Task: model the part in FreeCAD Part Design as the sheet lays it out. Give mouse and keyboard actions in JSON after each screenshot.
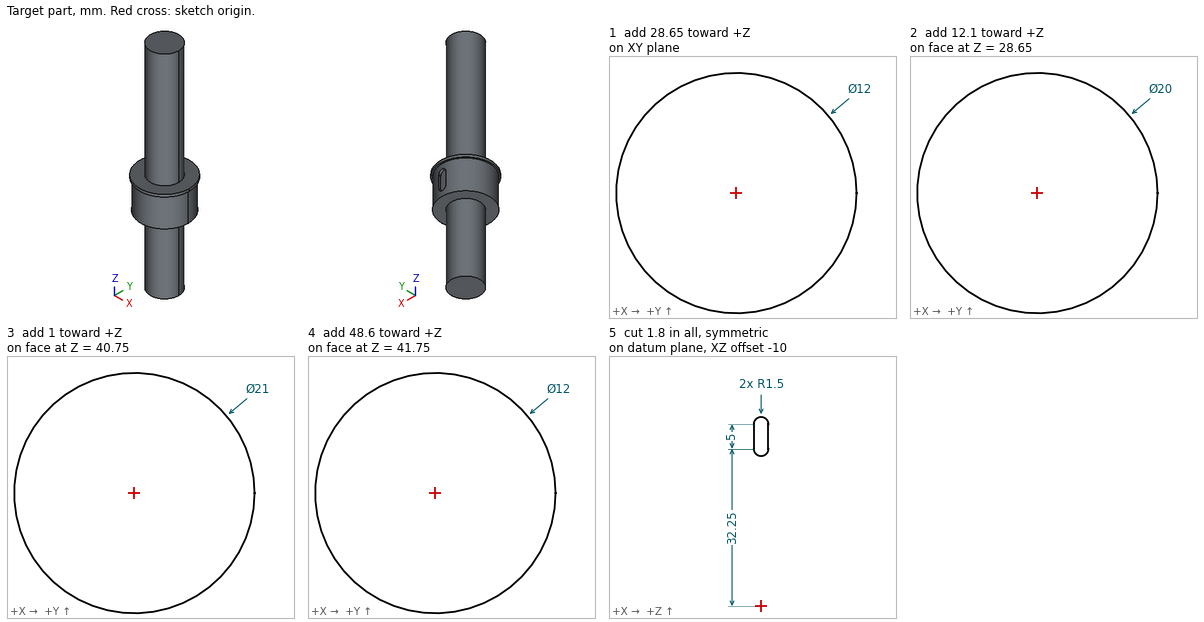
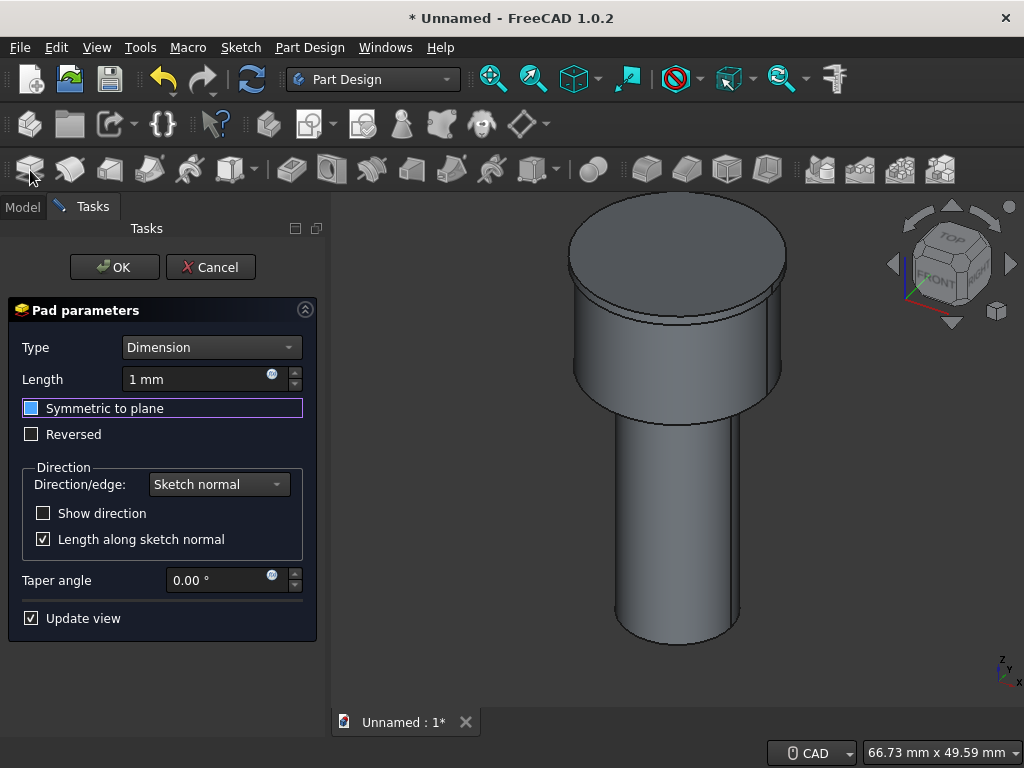
{"action": "left_click", "coordinate": [115, 267]}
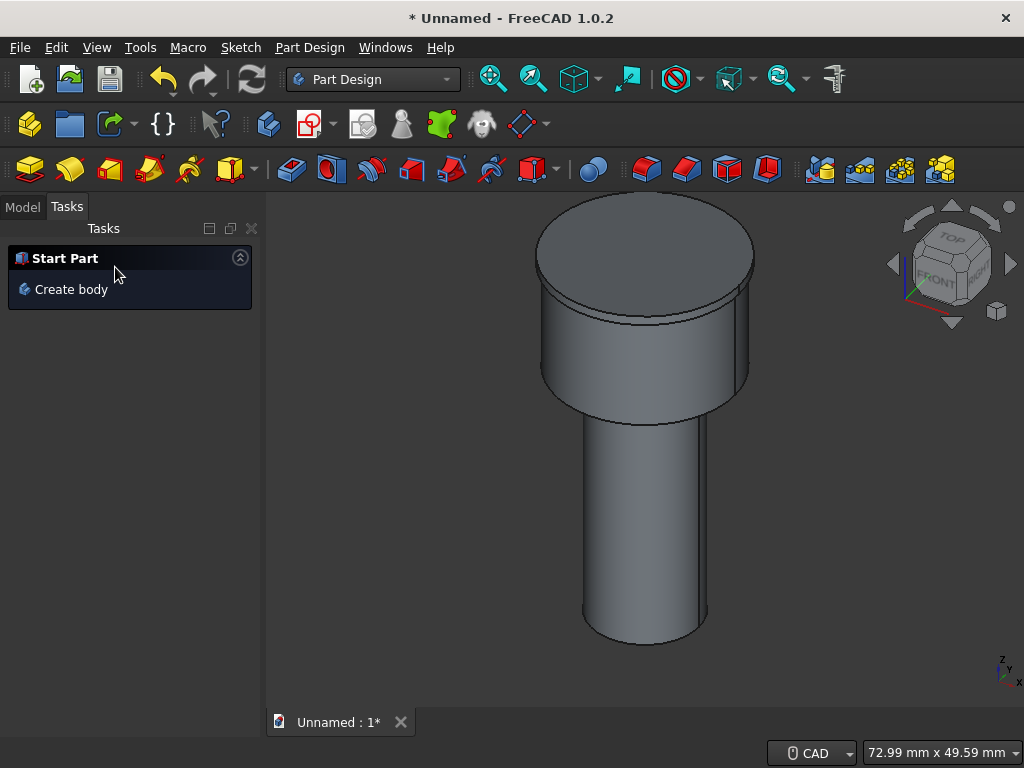
{"action": "left_click", "coordinate": [494, 80]}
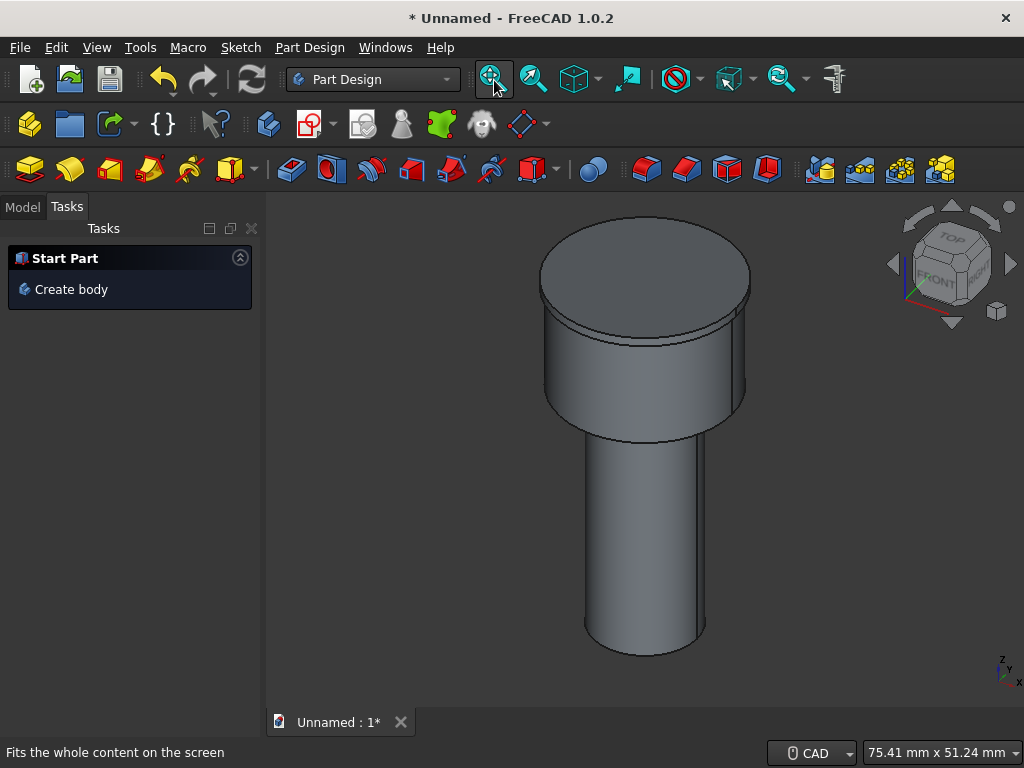
{"action": "left_click", "coordinate": [645, 277]}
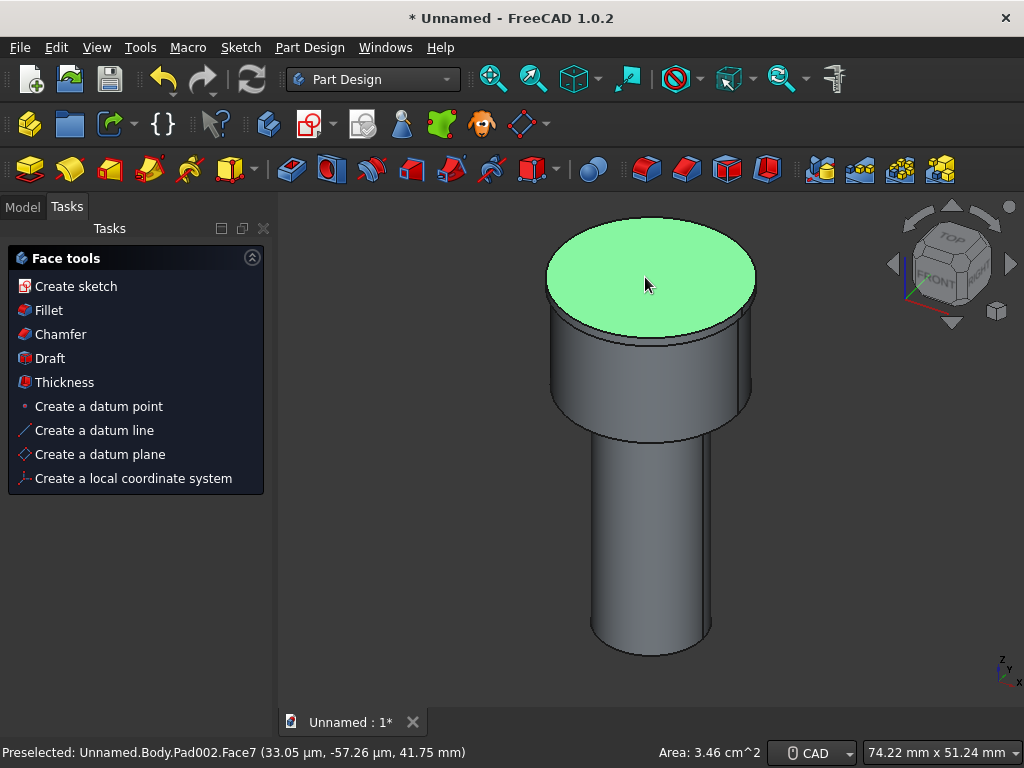
{"action": "left_click", "coordinate": [310, 124]}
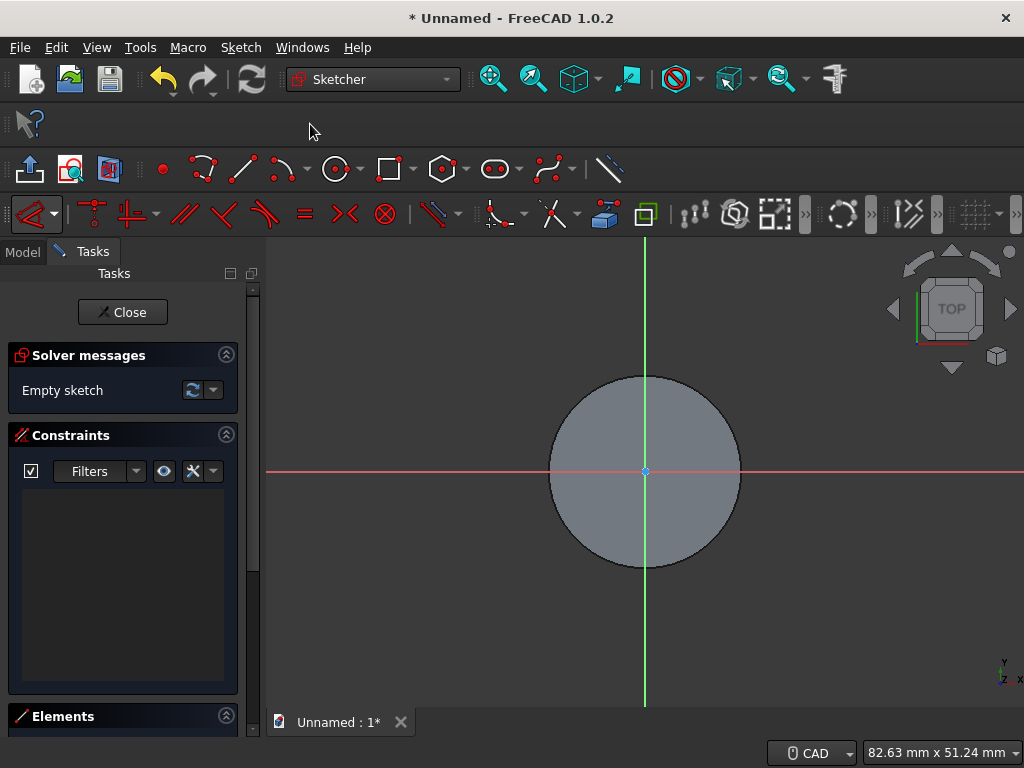
{"action": "scroll", "coordinate": [685, 472], "scroll_direction": "up", "scroll_amount": 5}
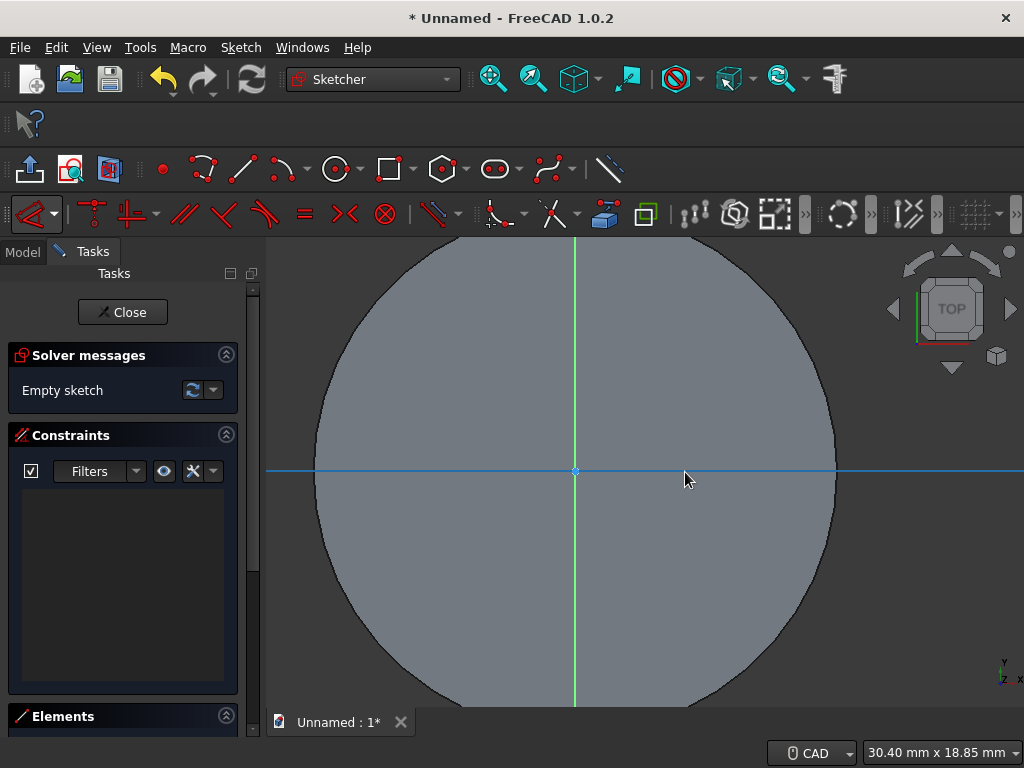
{"action": "left_click", "coordinate": [336, 170]}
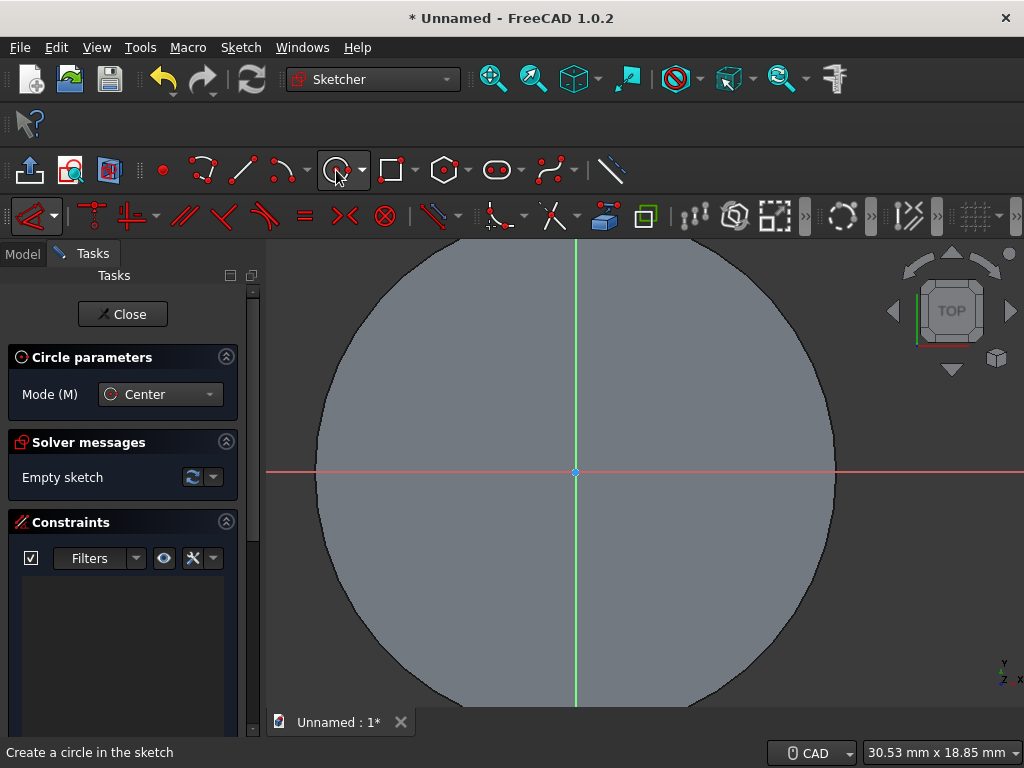
{"action": "left_click", "coordinate": [576, 472]}
{"action": "left_click", "coordinate": [681, 367]}
{"action": "key", "text": "Escape"}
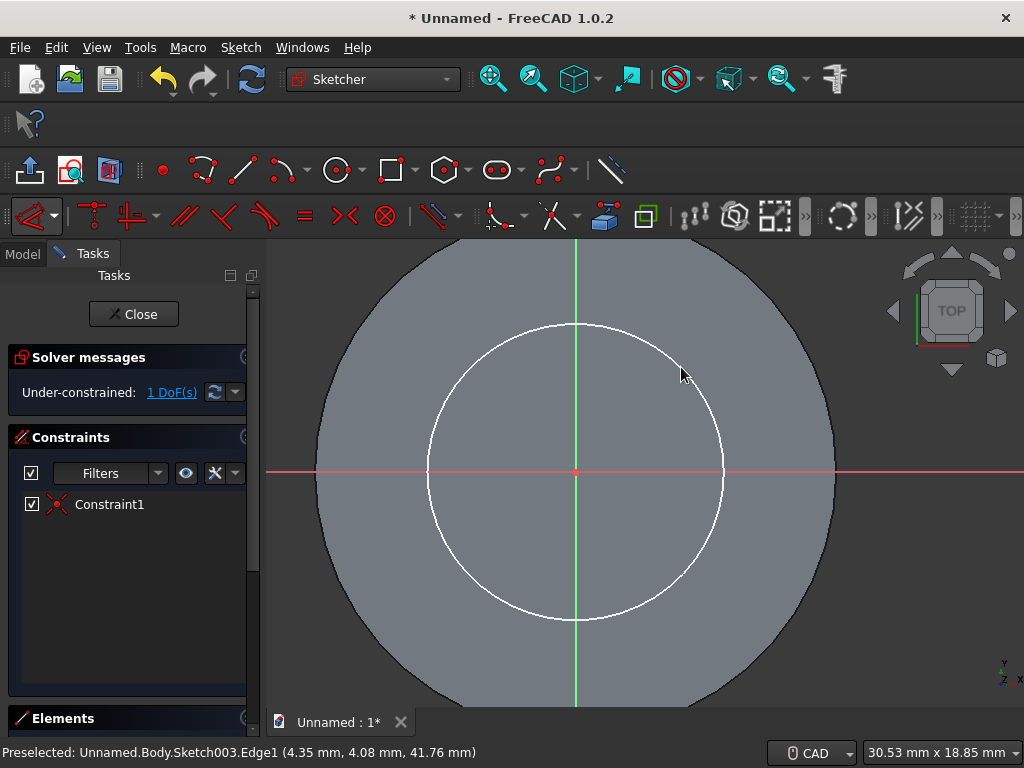
{"action": "left_click", "coordinate": [680, 367]}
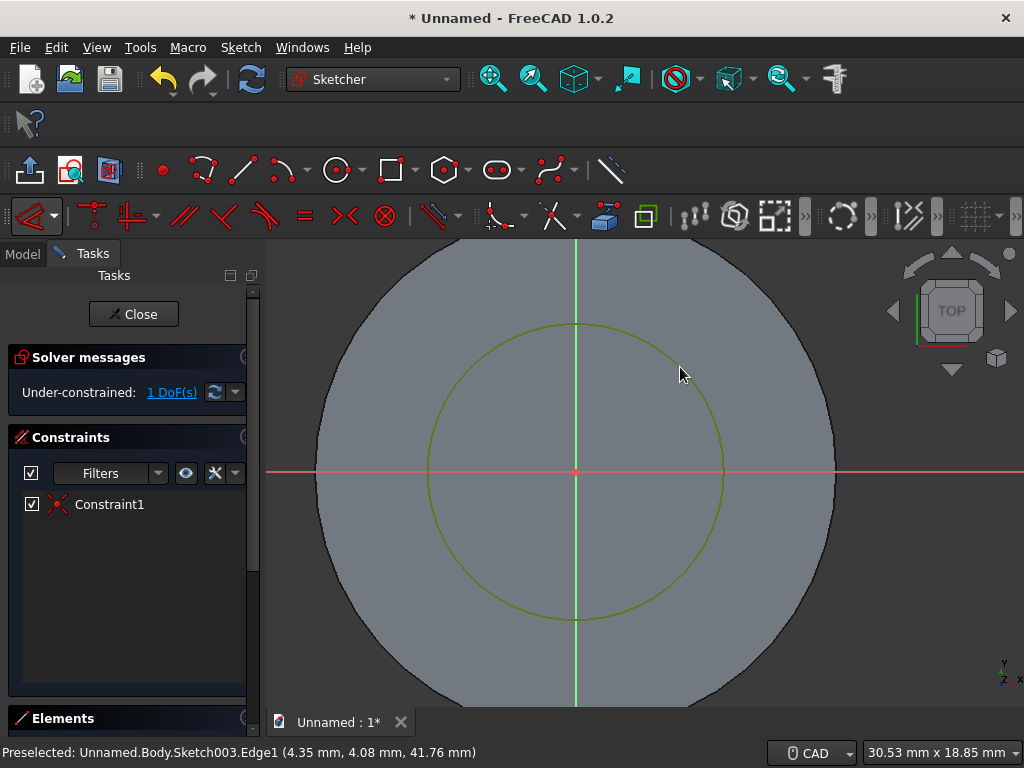
{"action": "key", "text": "k o"}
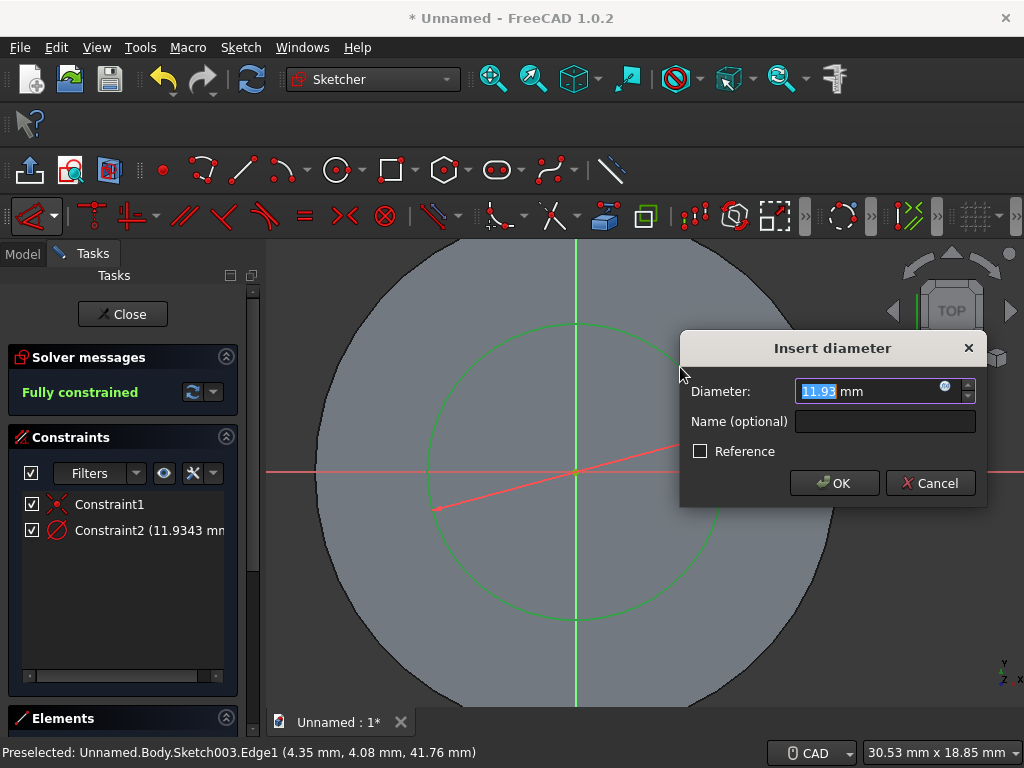
{"action": "type", "text": "12"}
{"action": "key", "text": "Return"}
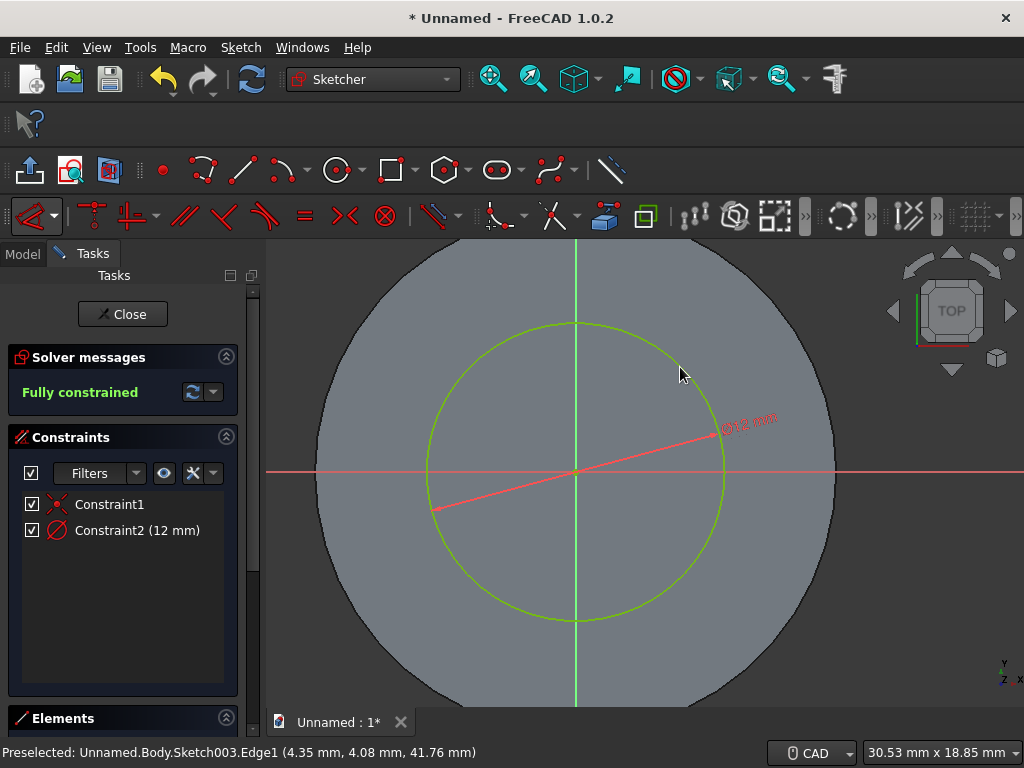
{"action": "left_click", "coordinate": [123, 314]}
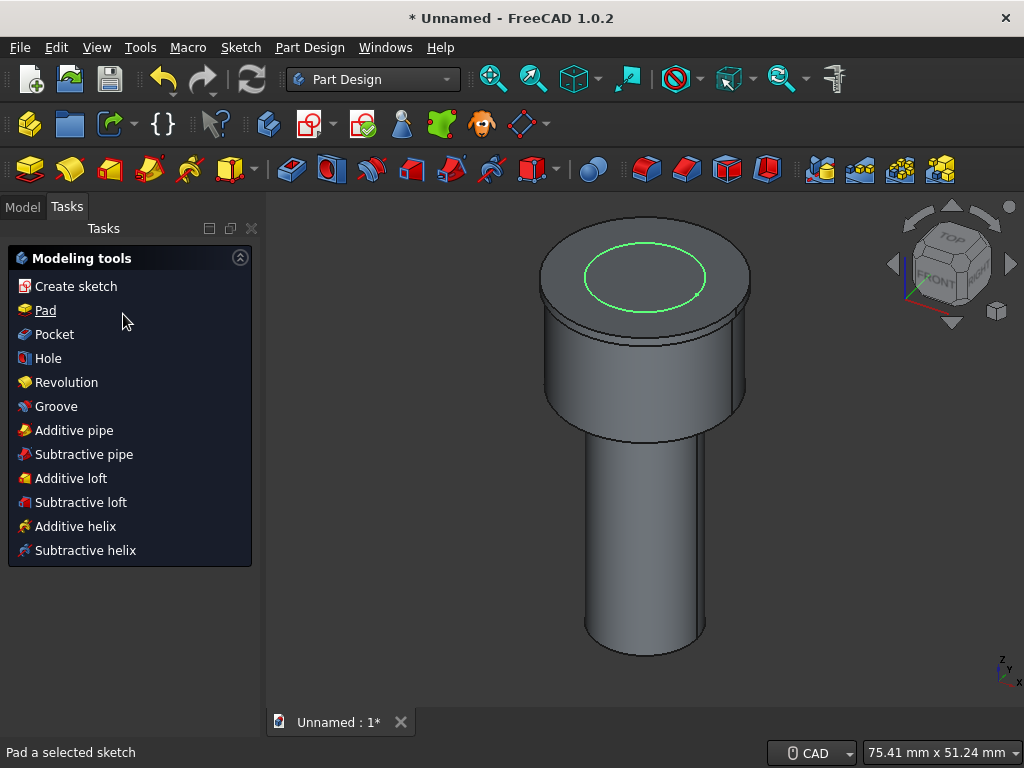
{"action": "left_click", "coordinate": [30, 170]}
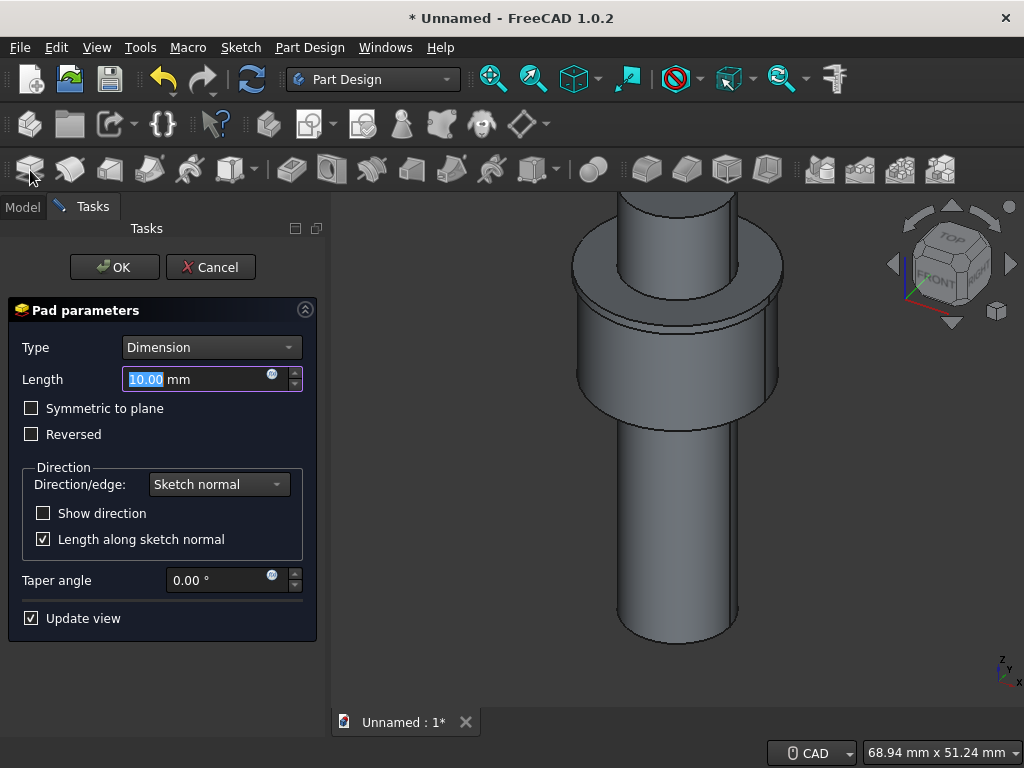
{"action": "type", "text": "48.6"}
{"action": "key", "text": "Tab"}